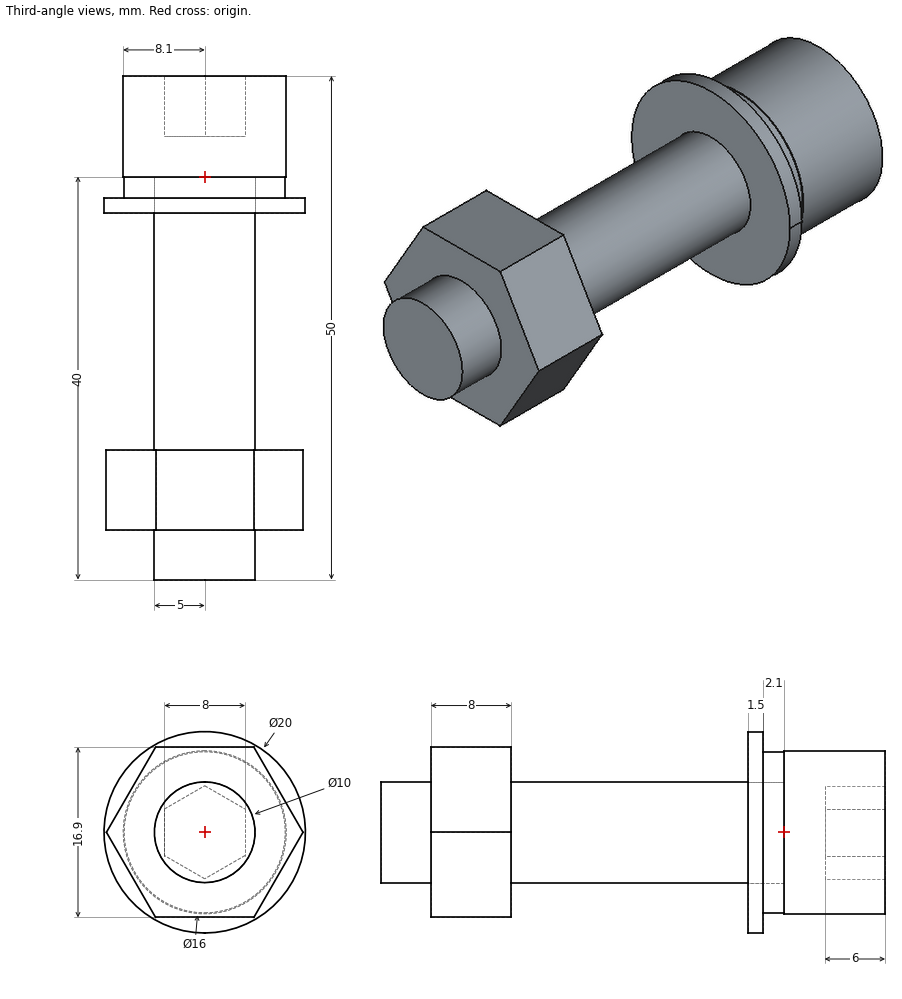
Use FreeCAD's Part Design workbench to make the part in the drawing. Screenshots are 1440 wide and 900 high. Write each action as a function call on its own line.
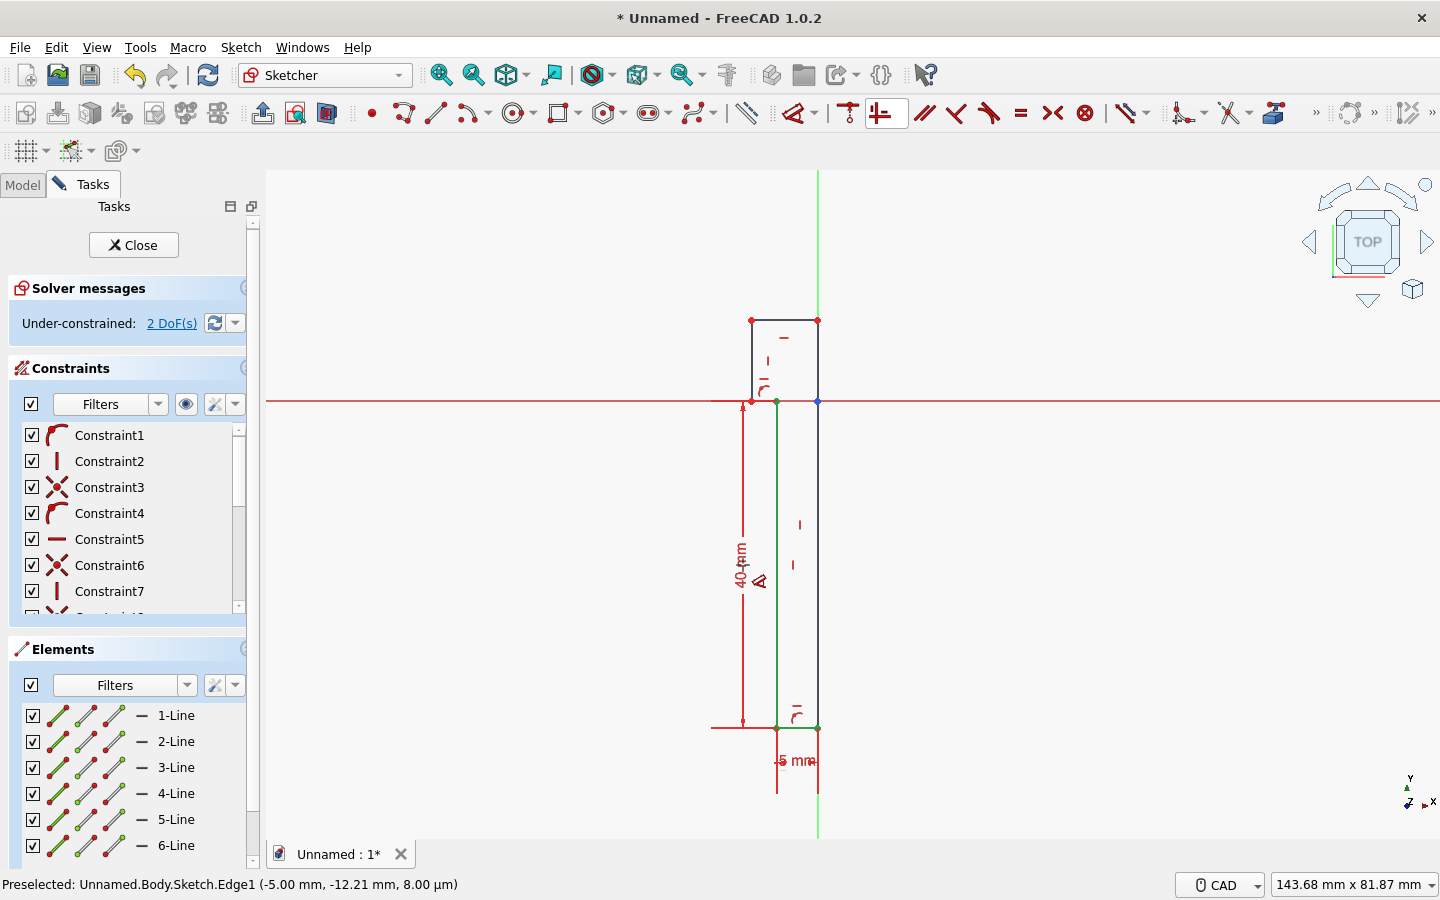
click(818, 606)
click(852, 524)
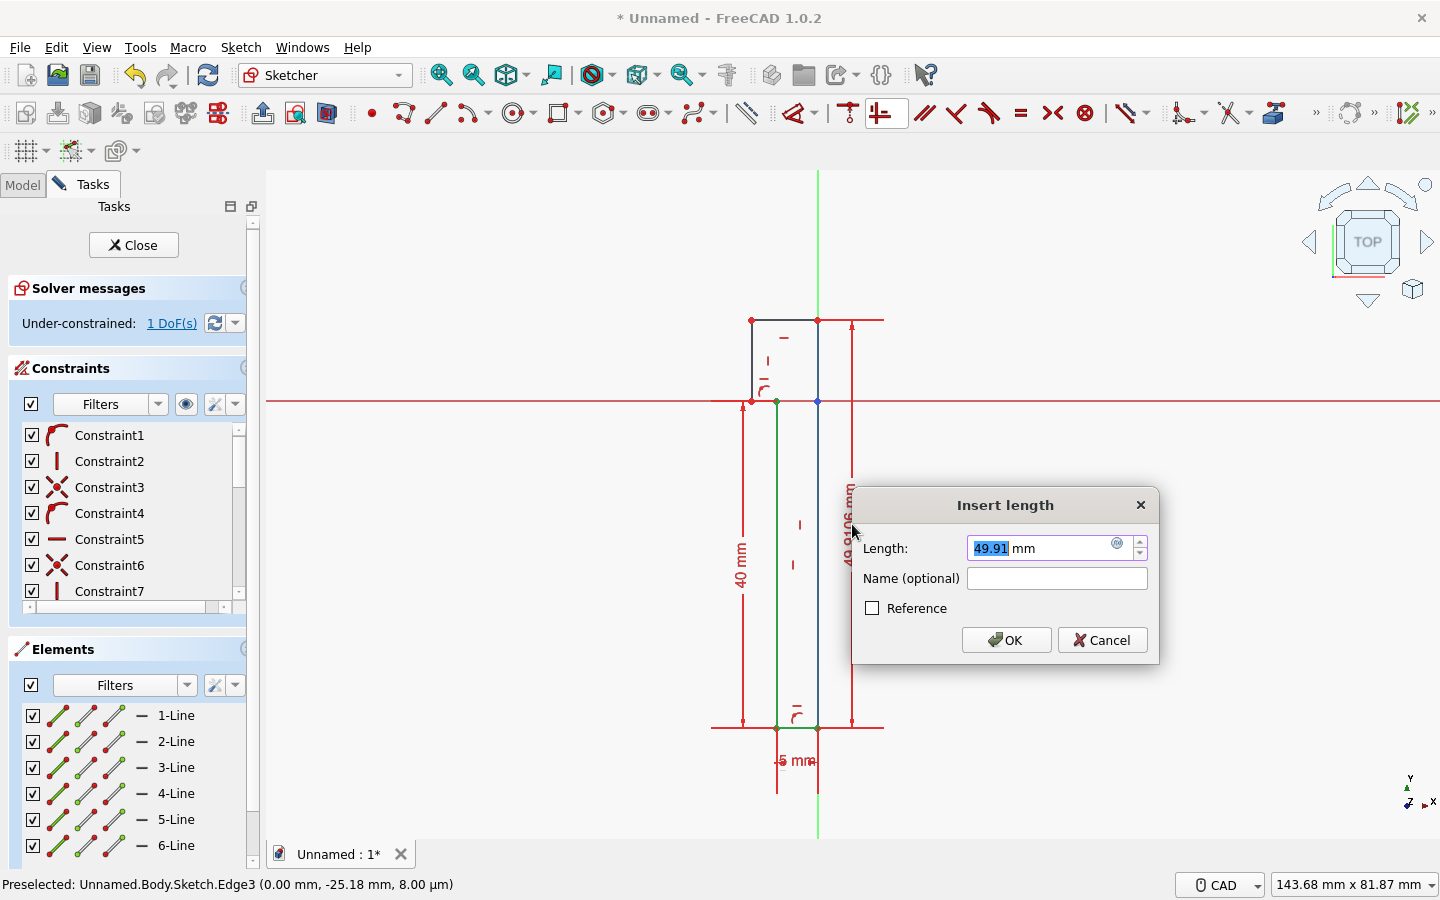
text(50)
key(Return)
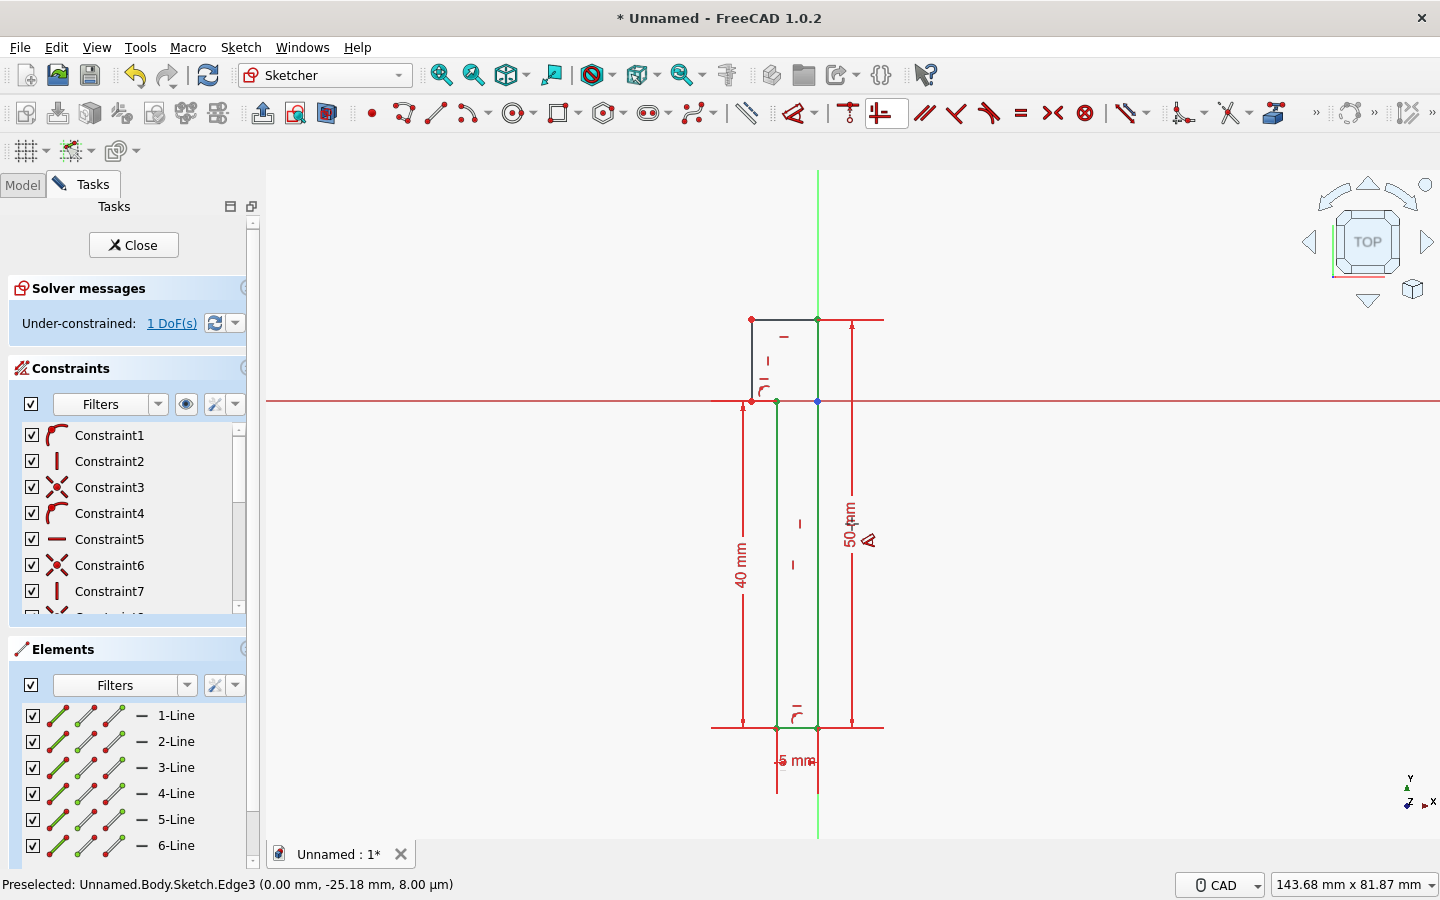
click(798, 320)
click(785, 286)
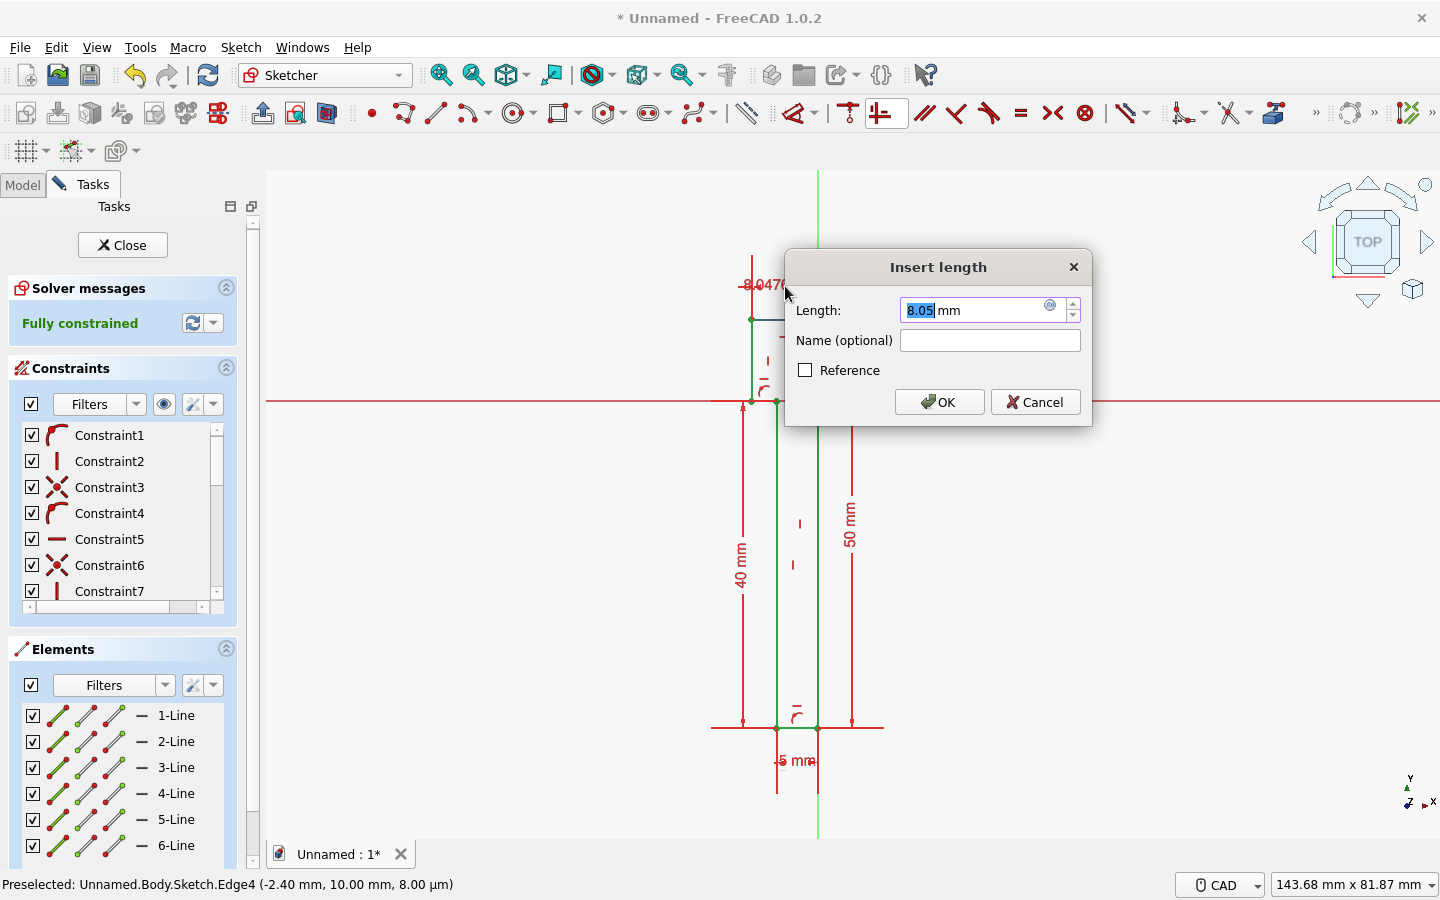
text(8.1)
key(Return)
key(Escape)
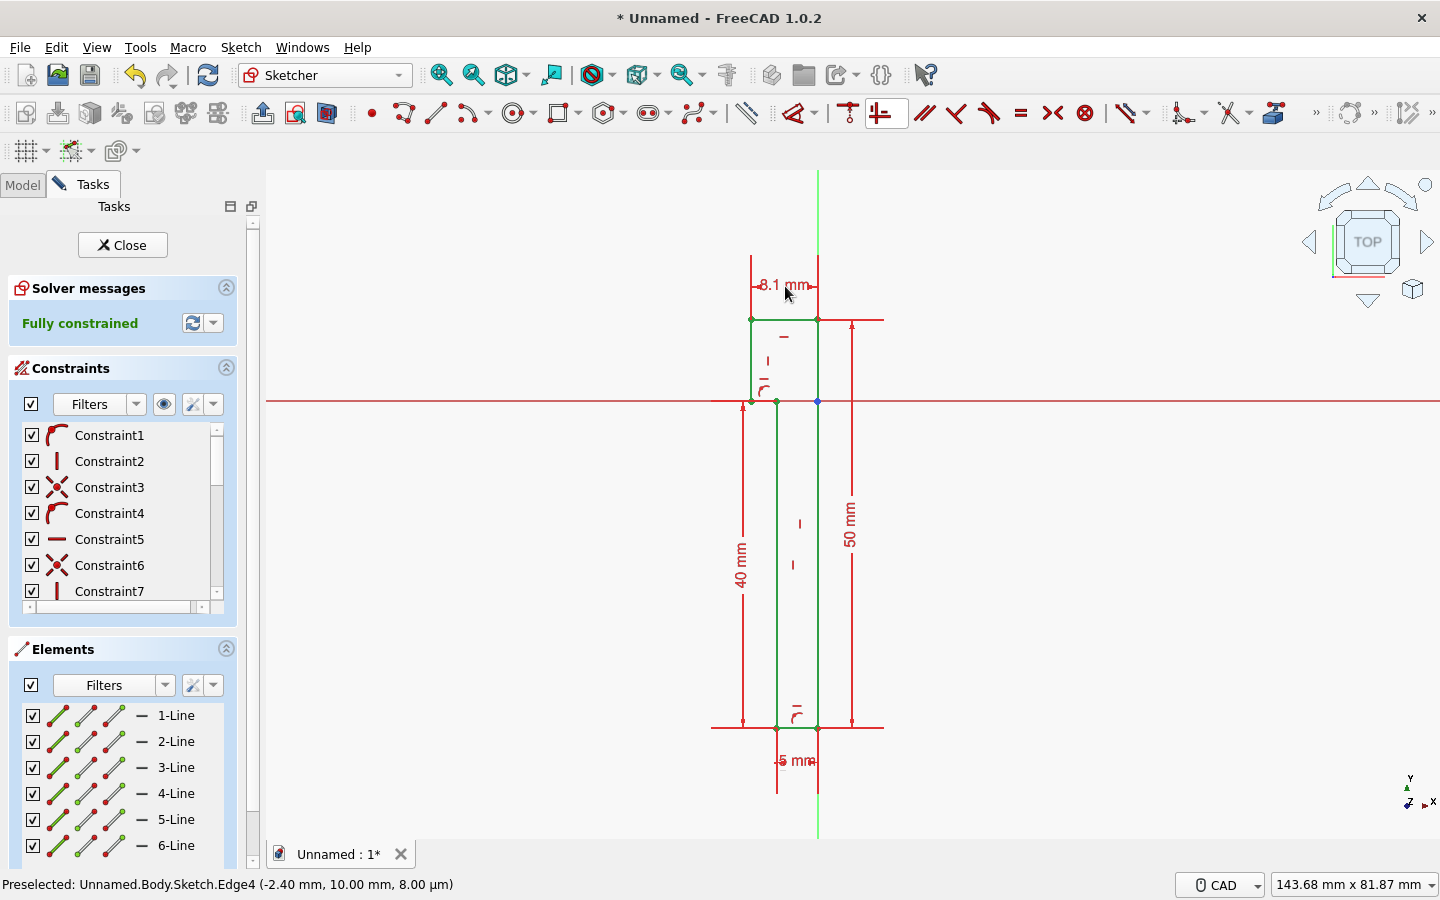
click(123, 245)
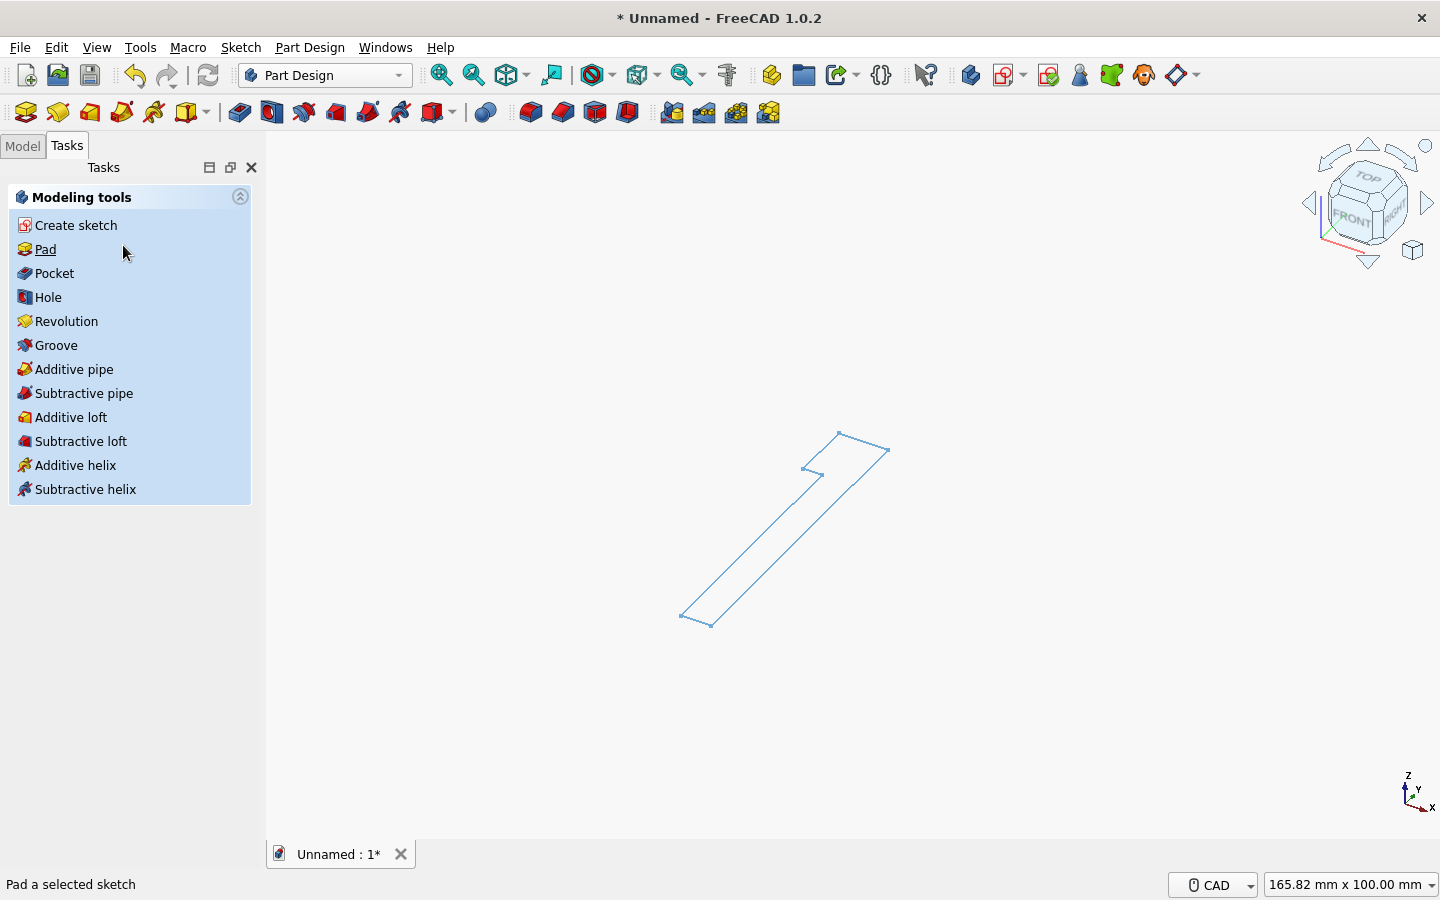
click(58, 112)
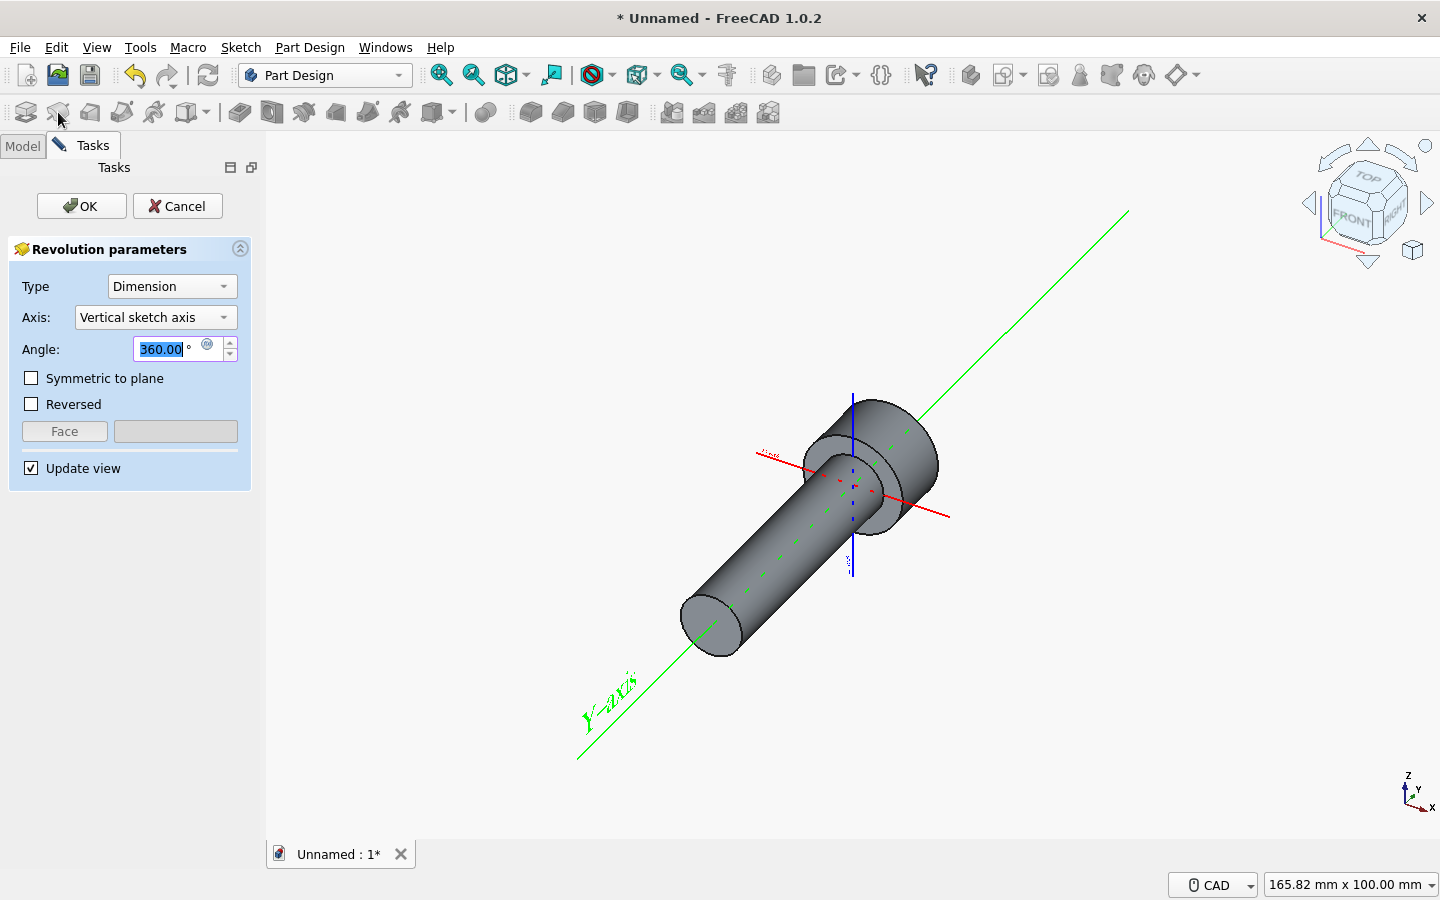
click(82, 206)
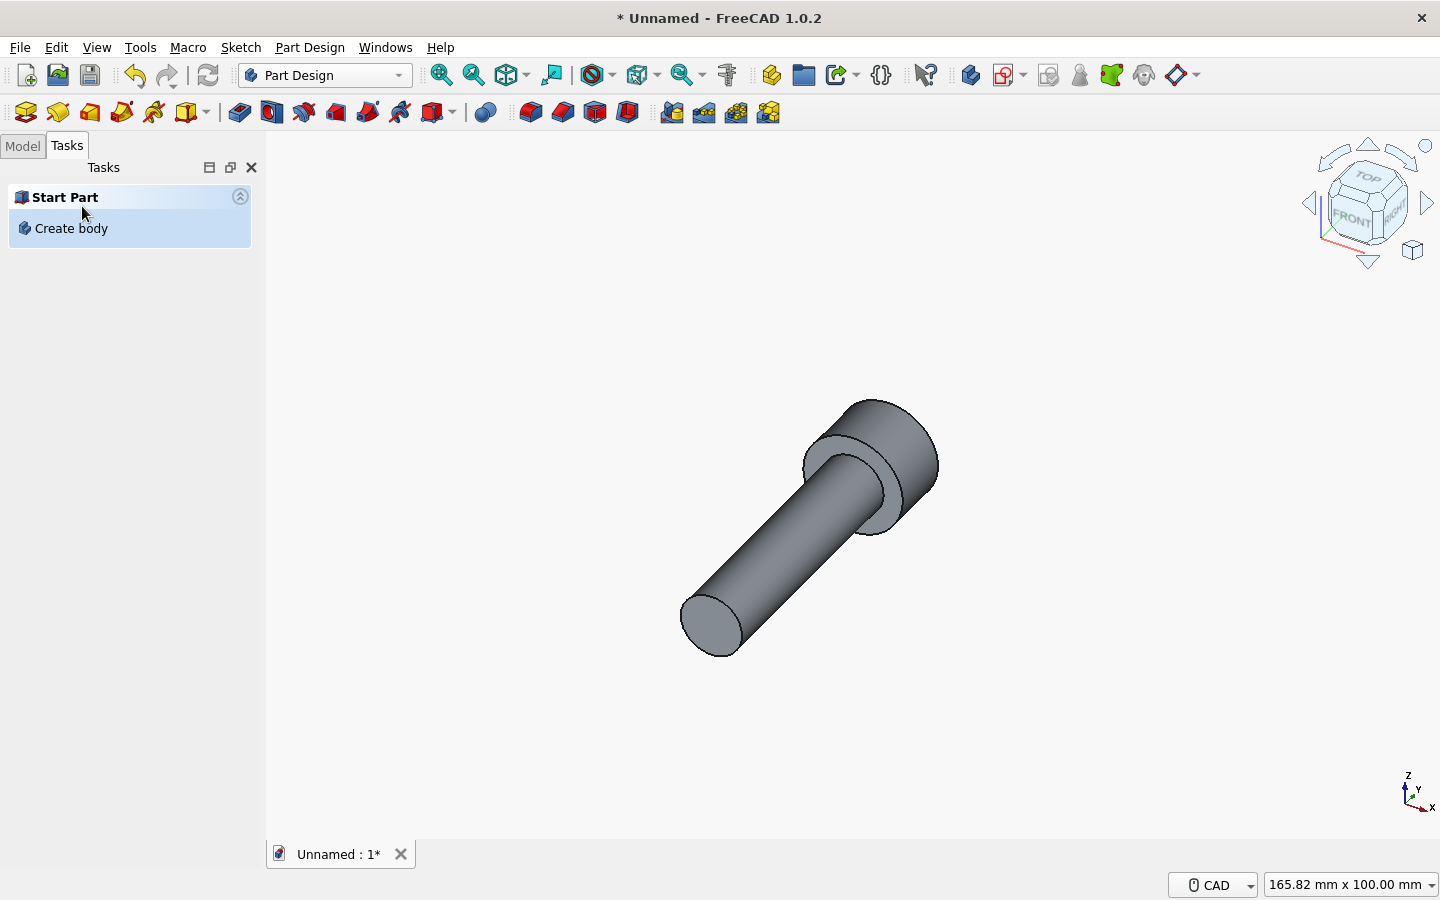
click(442, 76)